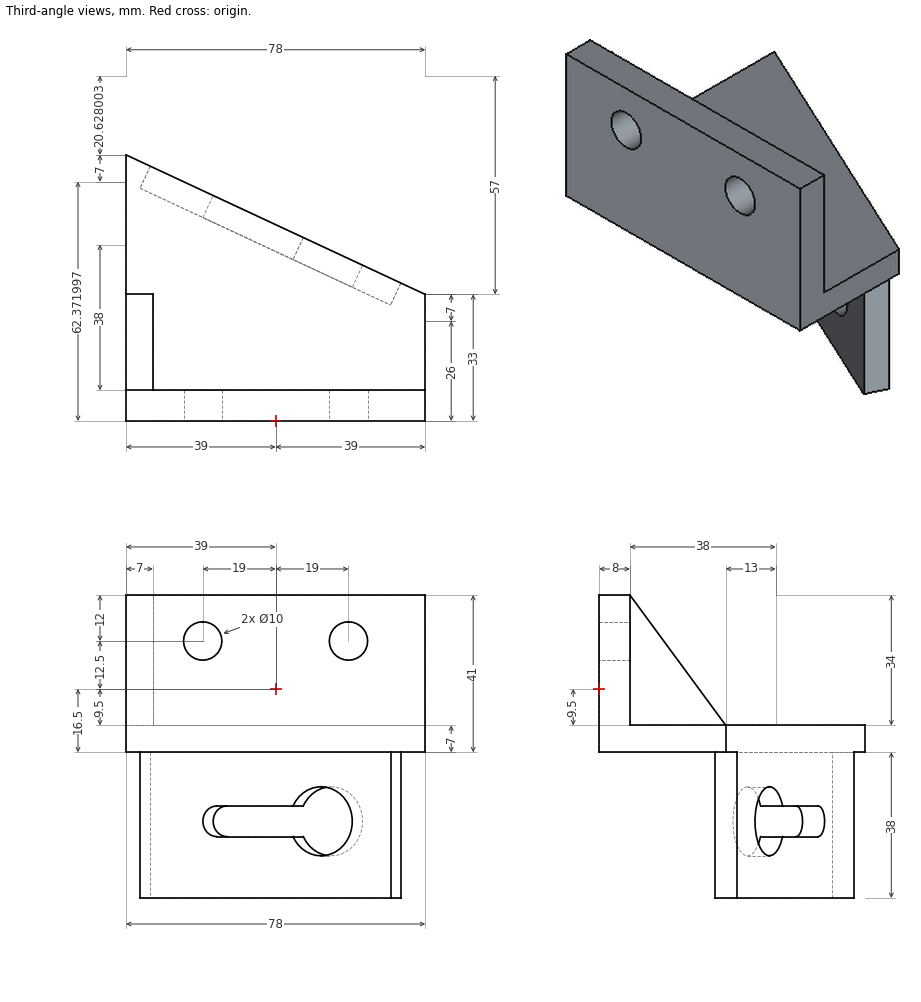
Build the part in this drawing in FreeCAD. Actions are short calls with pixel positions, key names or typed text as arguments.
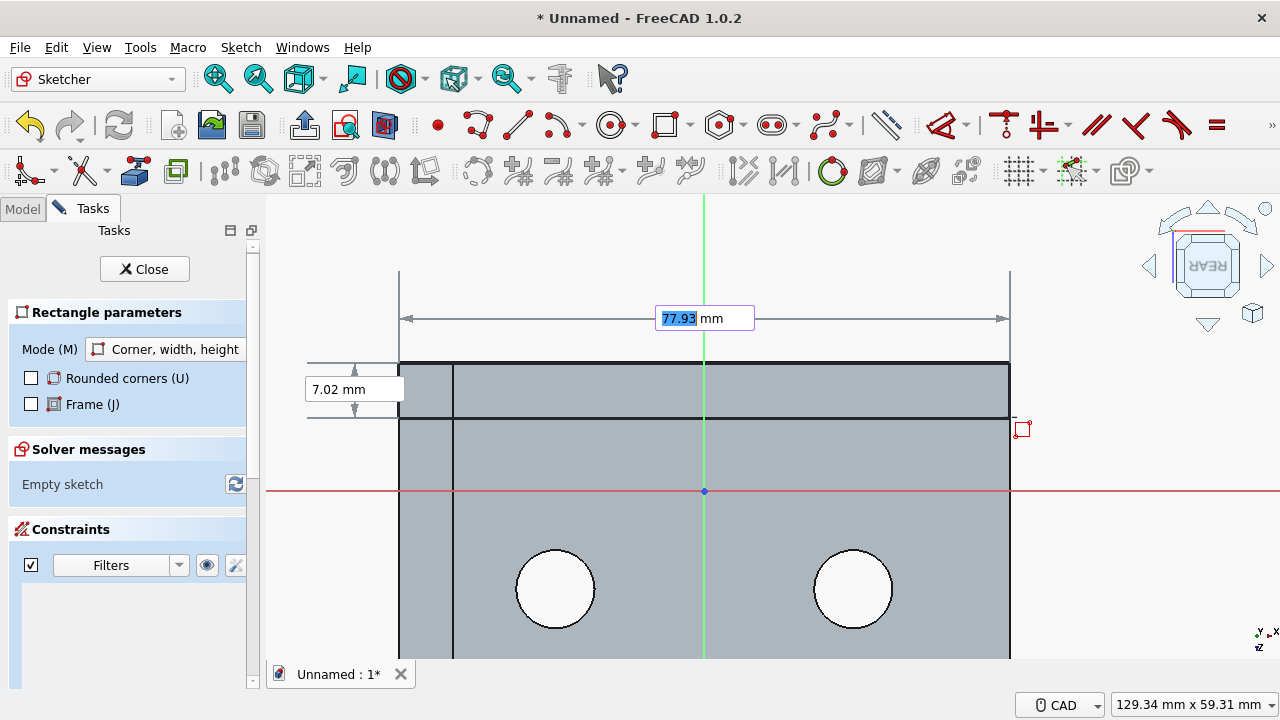
text(78)
key(Tab)
text(7)
key(Return)
key(Escape)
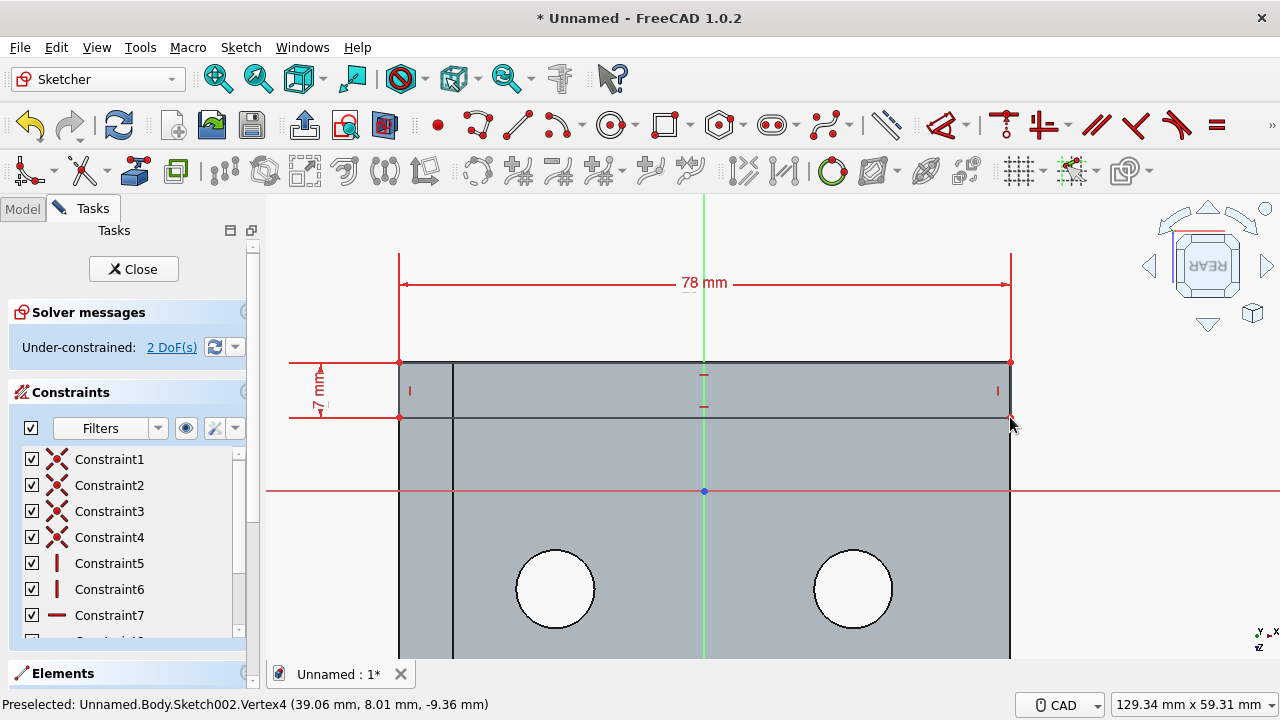
click(942, 126)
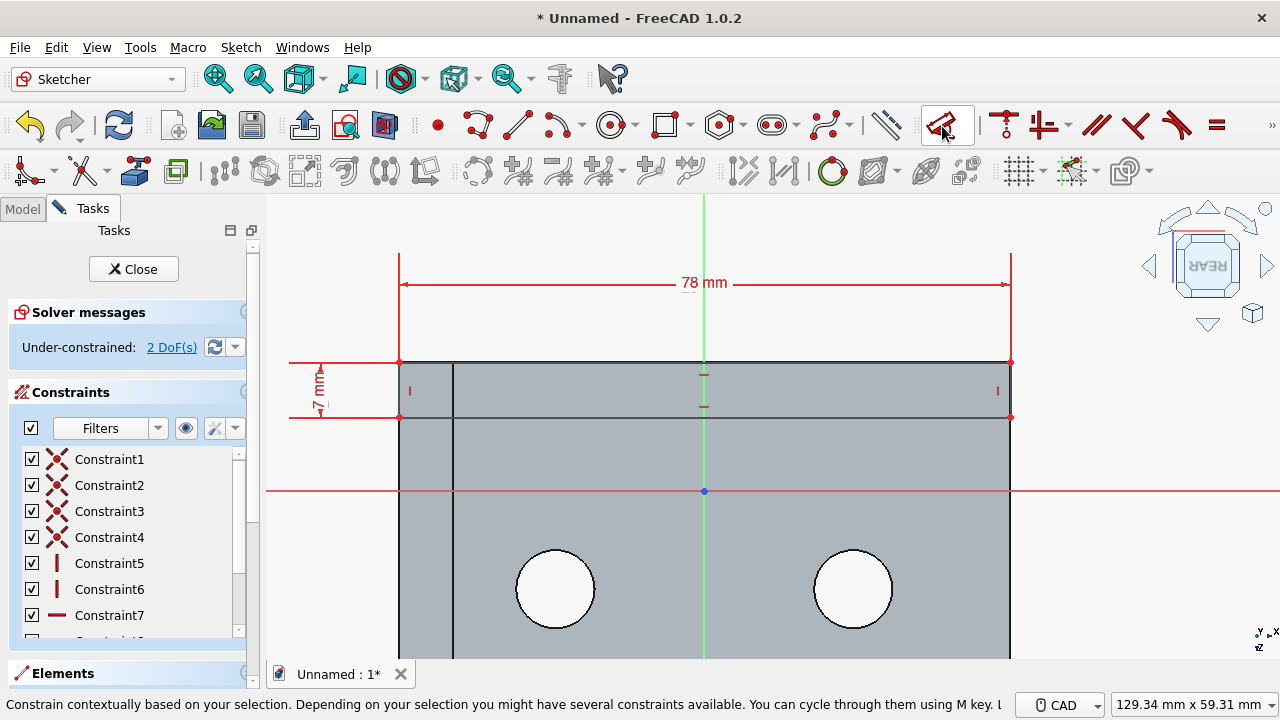
click(399, 363)
click(552, 525)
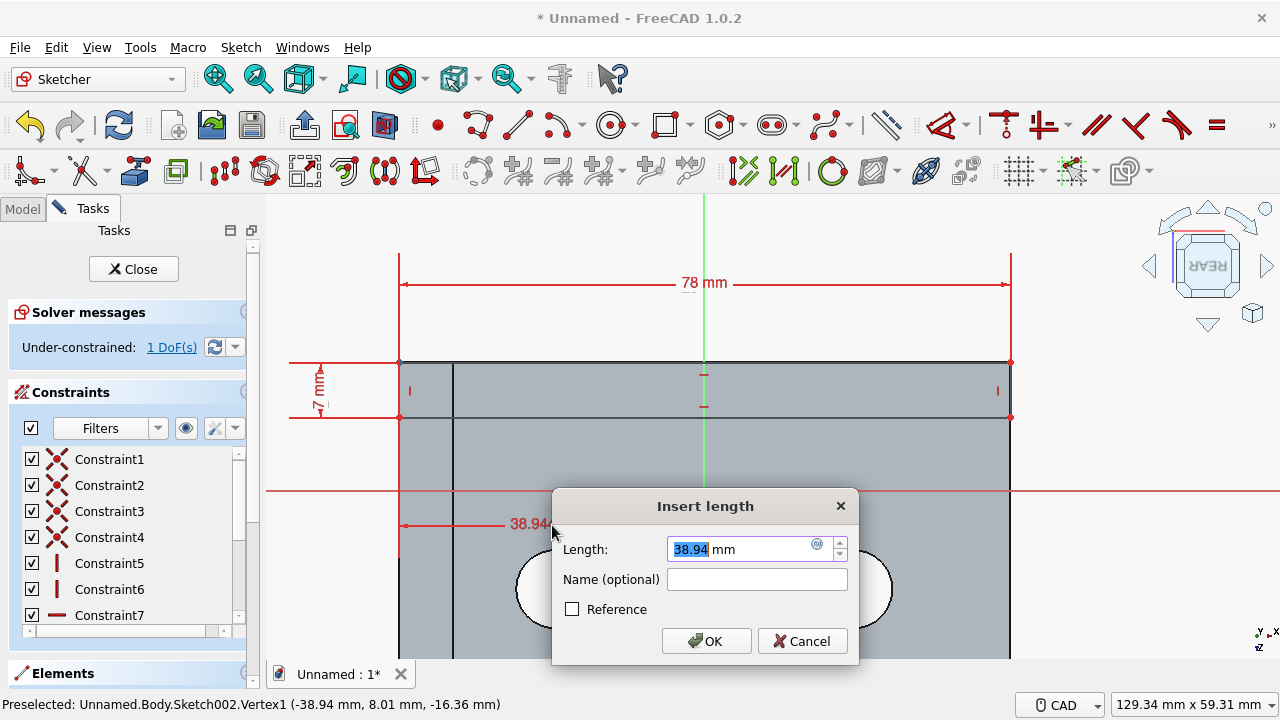
text(39)
key(Return)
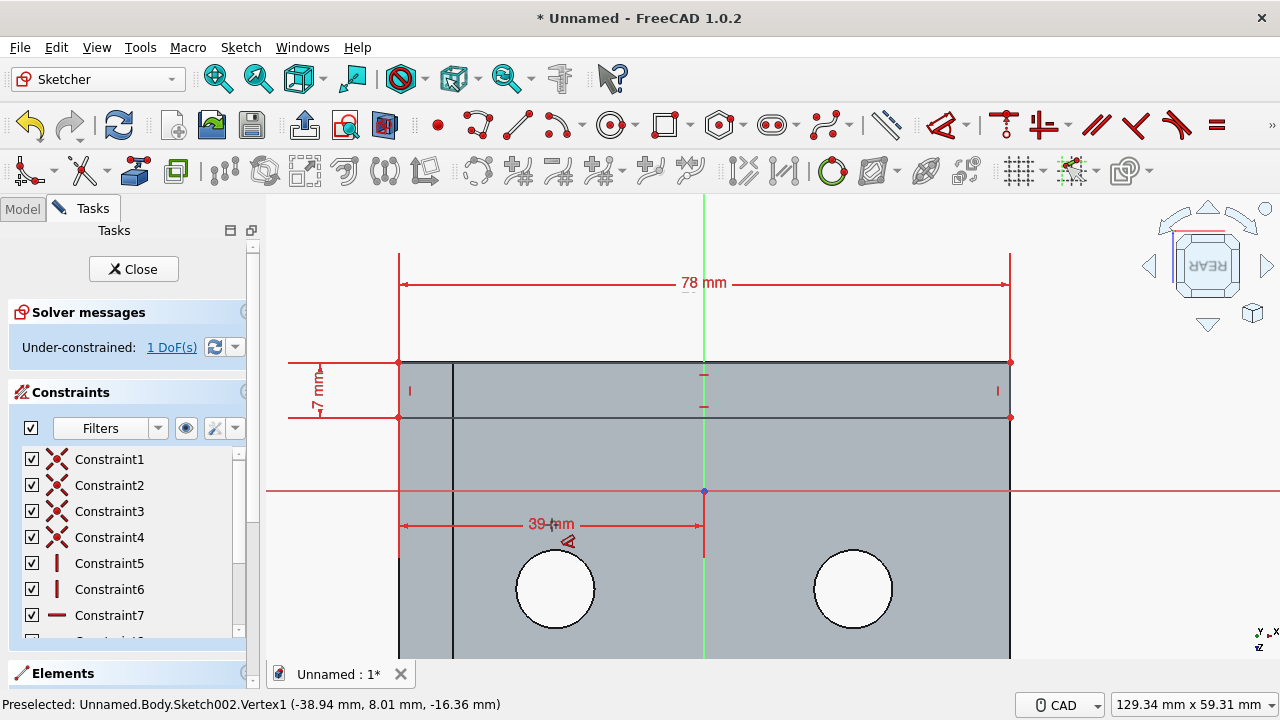
click(399, 418)
click(365, 455)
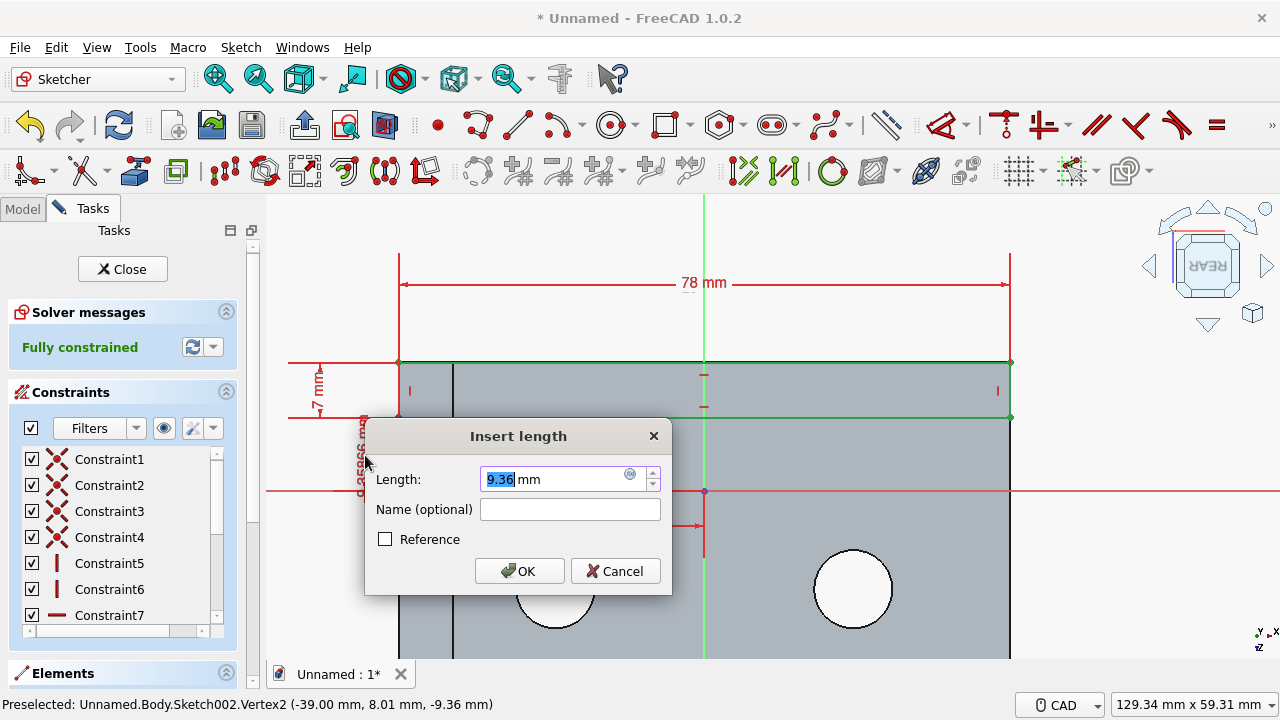
text(9.5)
key(Return)
key(Escape)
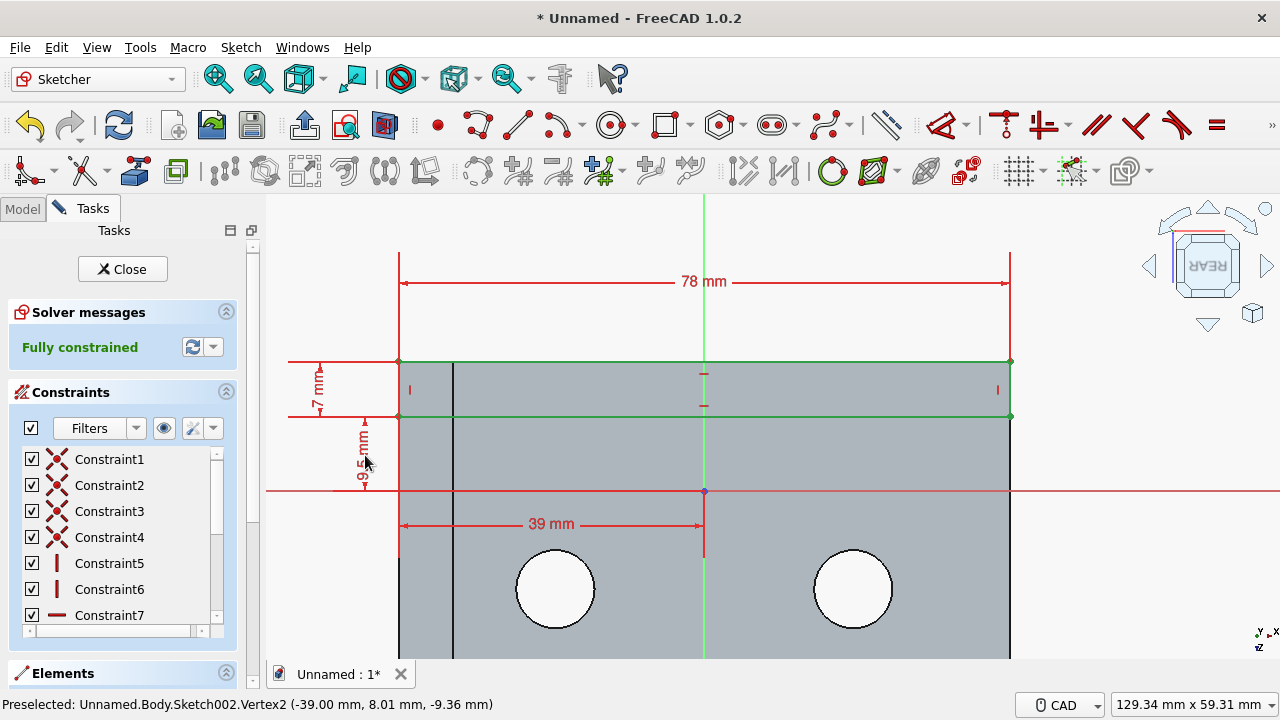
click(123, 269)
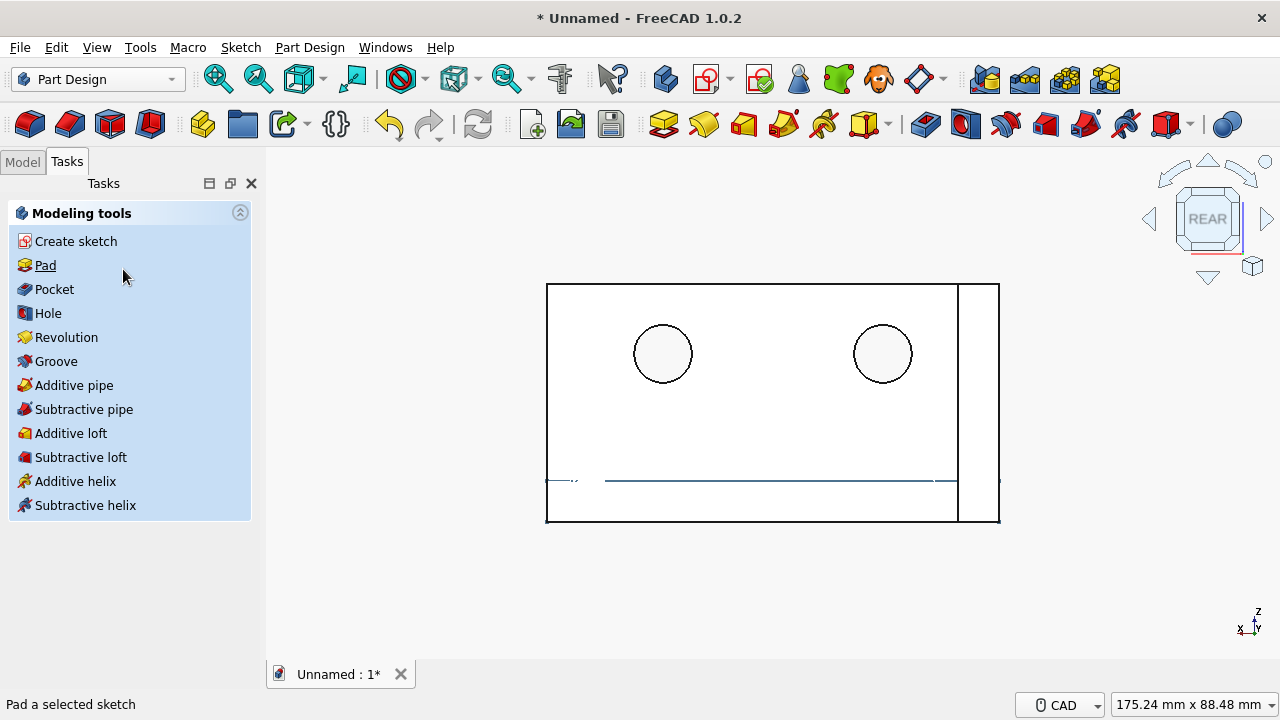
click(664, 124)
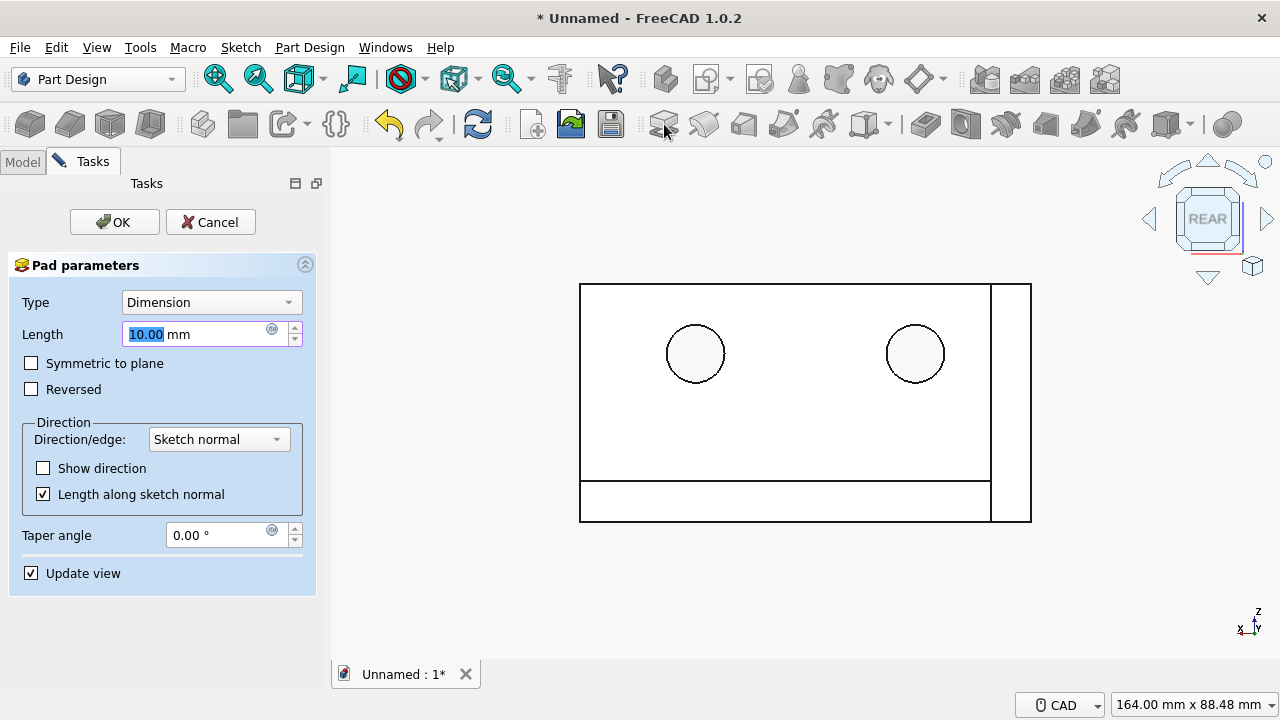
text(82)
key(Tab)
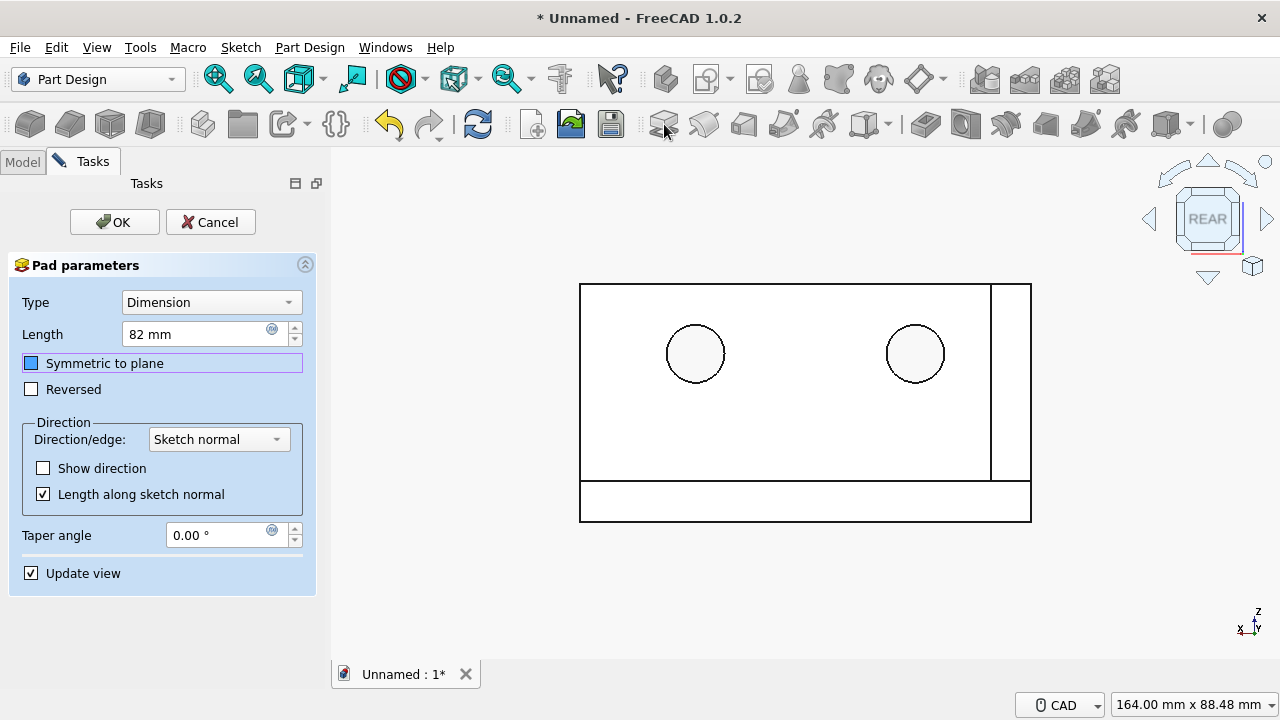
click(115, 222)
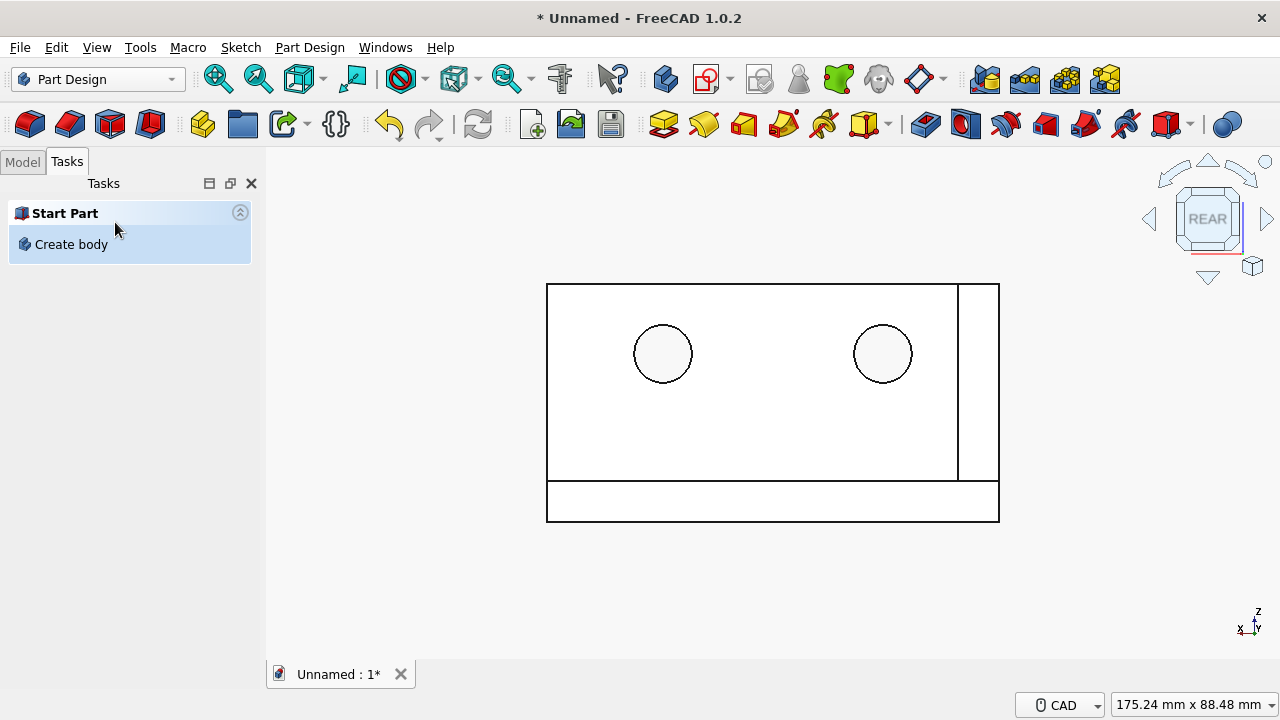
key(0)